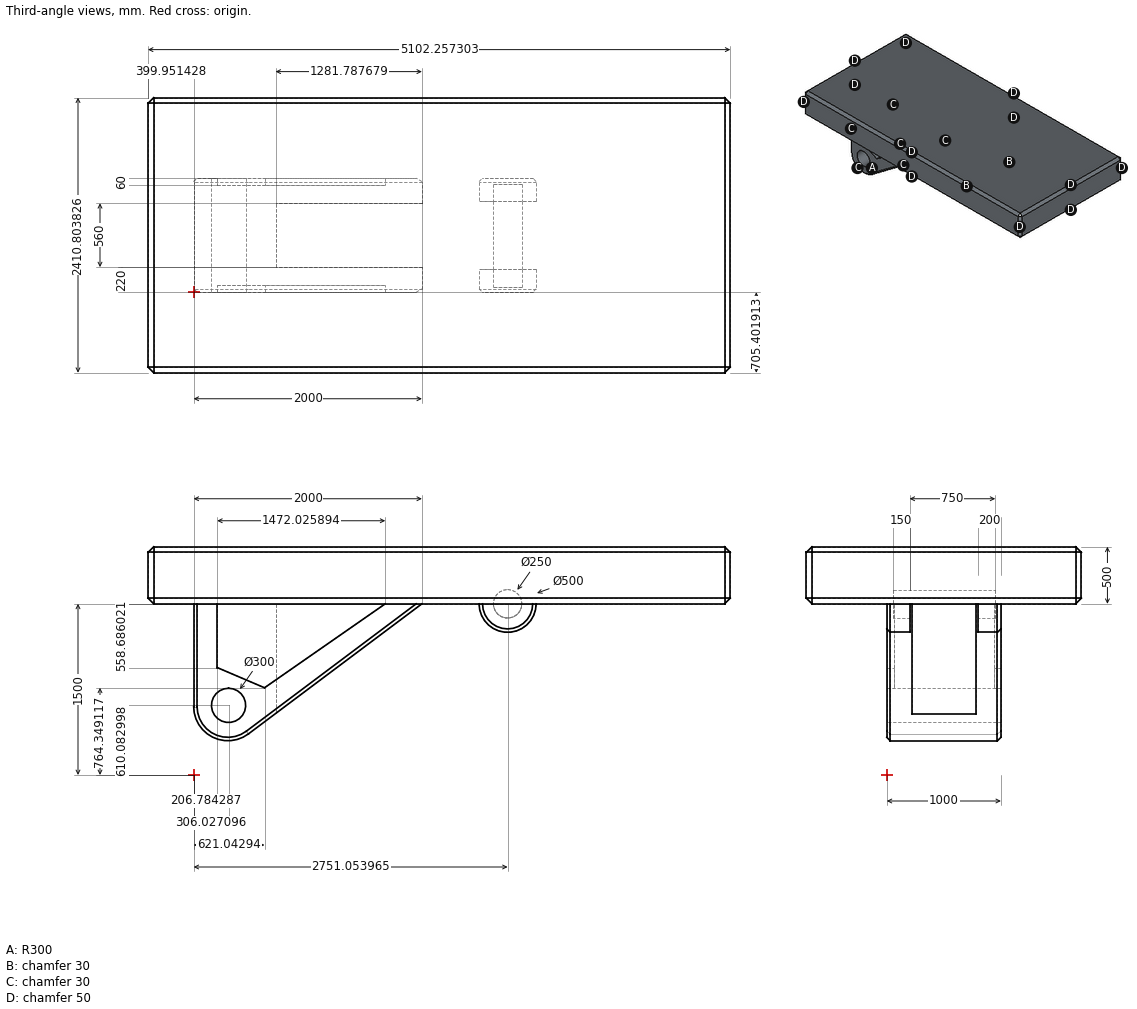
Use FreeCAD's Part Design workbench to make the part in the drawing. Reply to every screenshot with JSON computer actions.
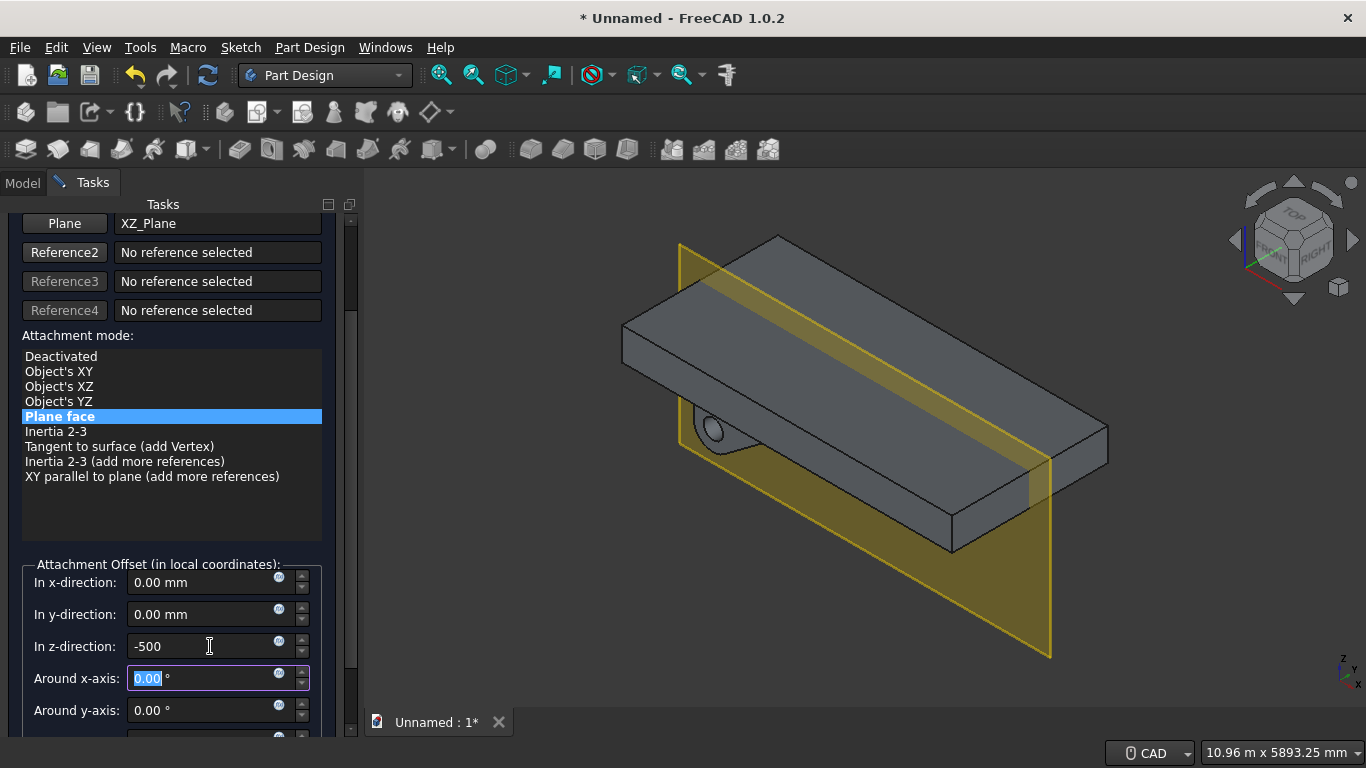
{"action": "scroll", "coordinate": [351, 475], "scroll_direction": "up", "scroll_amount": 3}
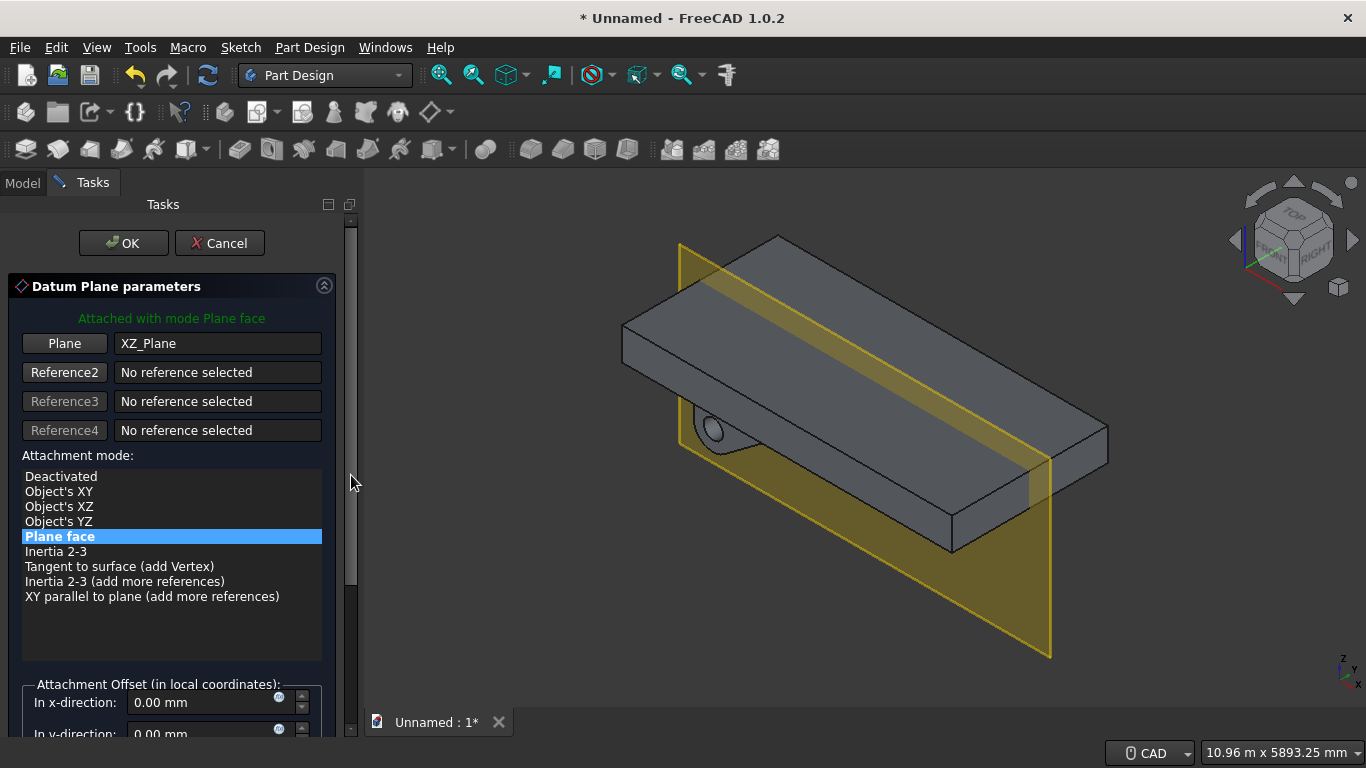
{"action": "left_click", "coordinate": [124, 243]}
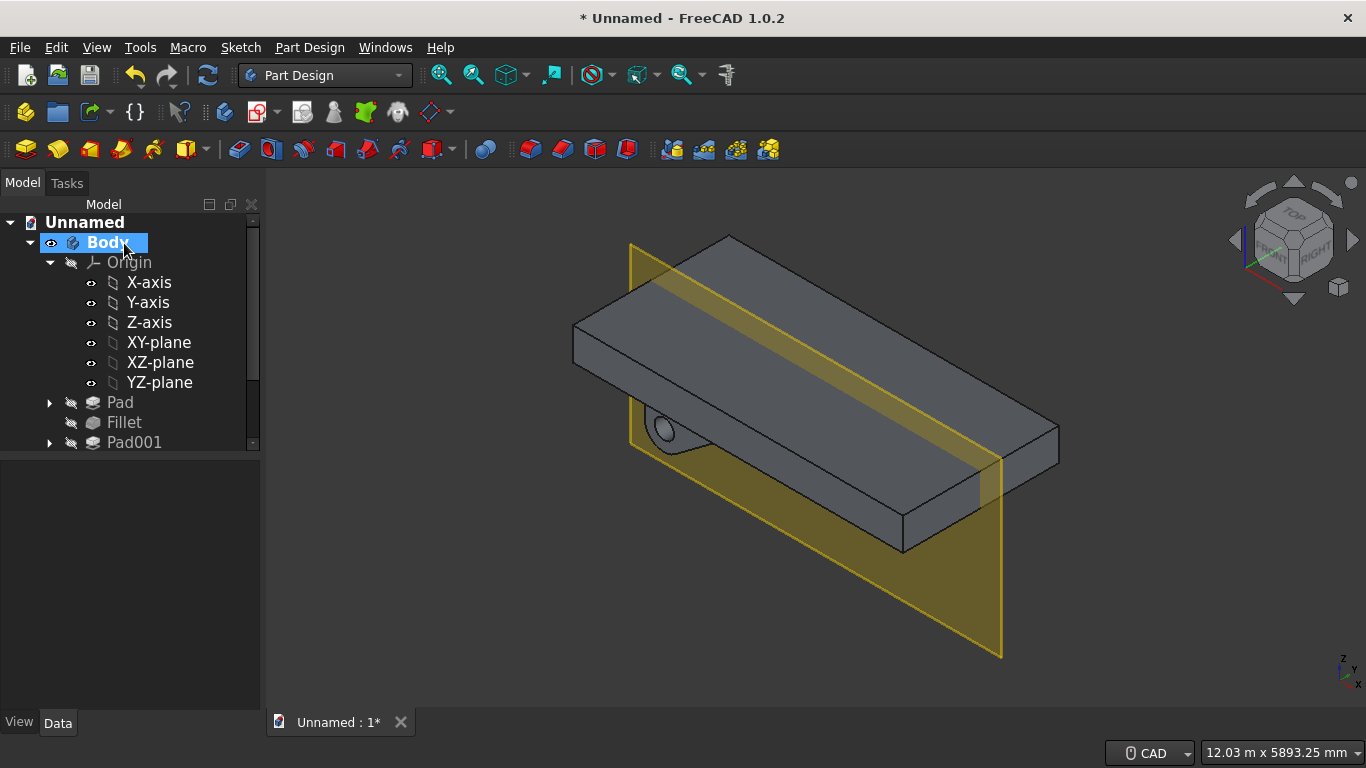
{"action": "scroll", "coordinate": [100, 338], "scroll_direction": "down", "scroll_amount": 3}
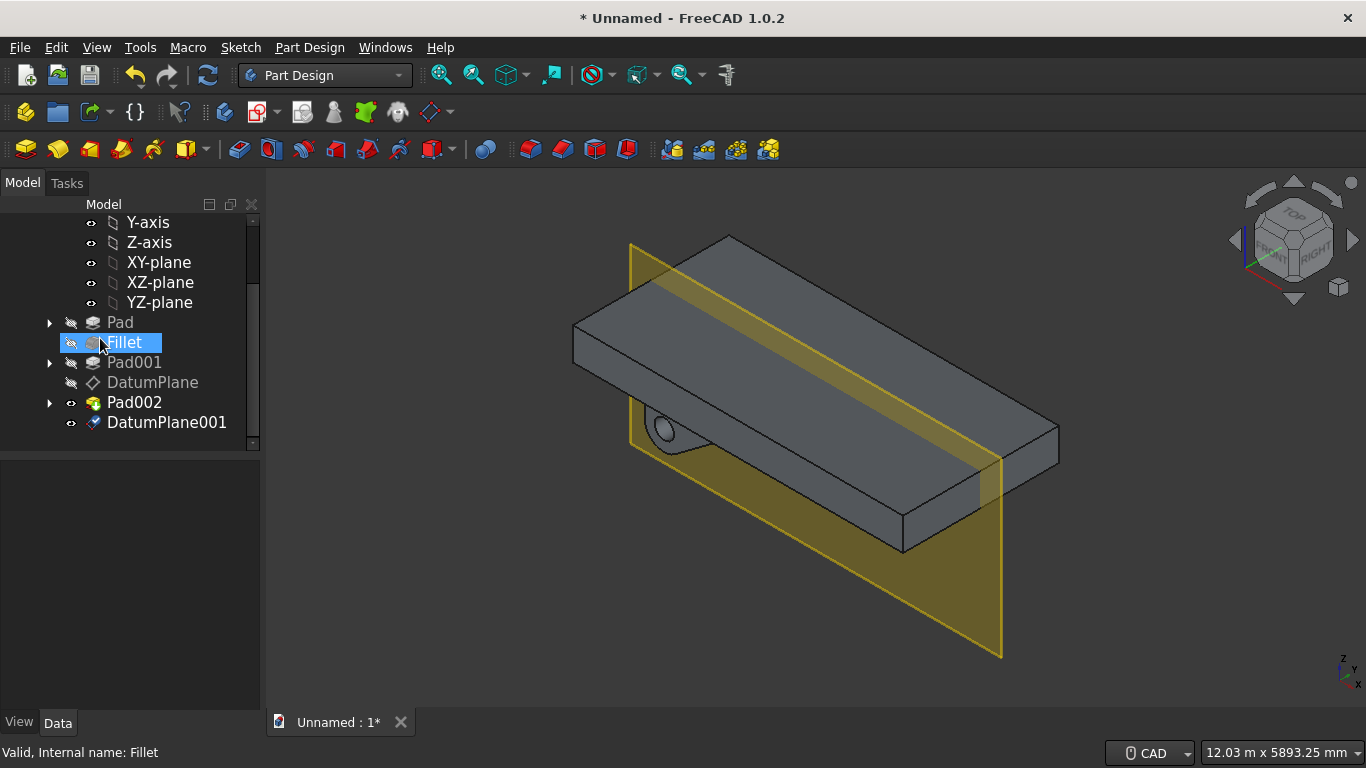
{"action": "left_click", "coordinate": [116, 403]}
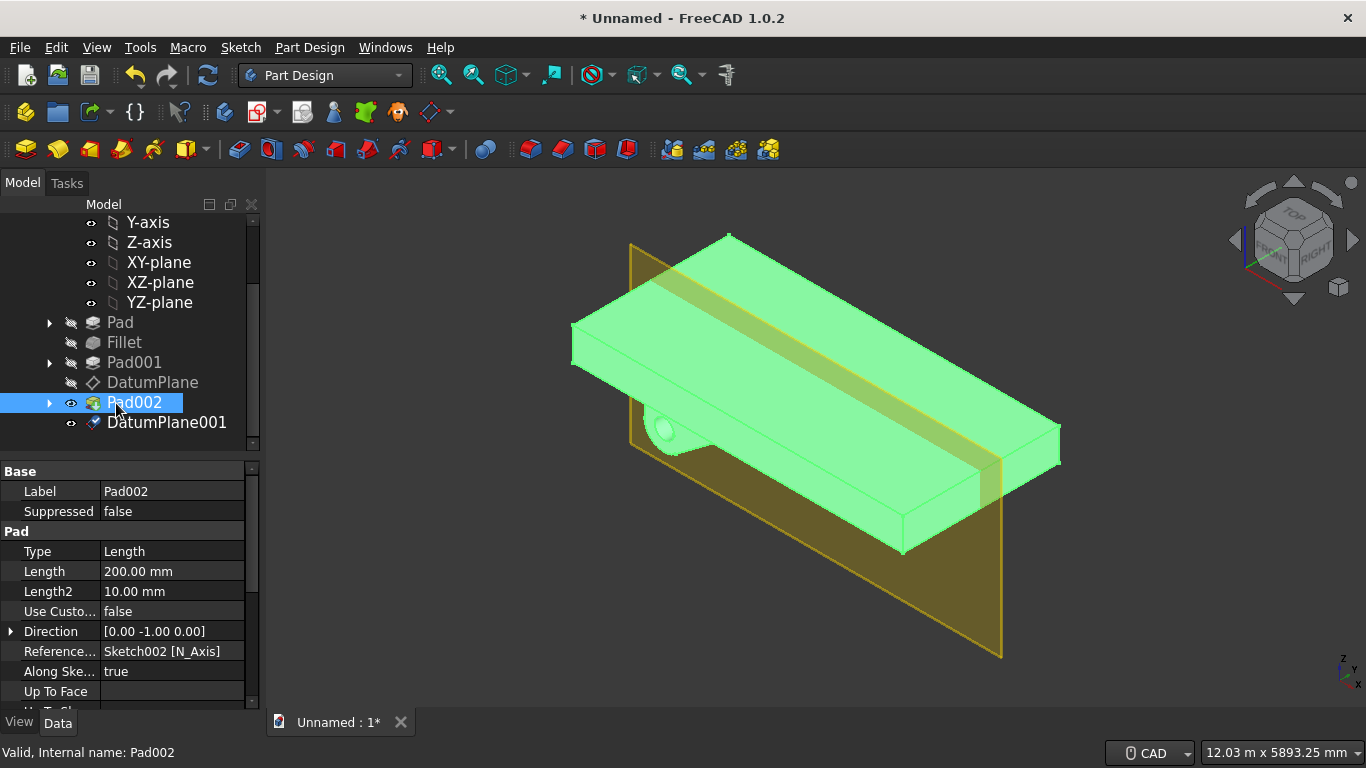
{"action": "left_click", "coordinate": [672, 150]}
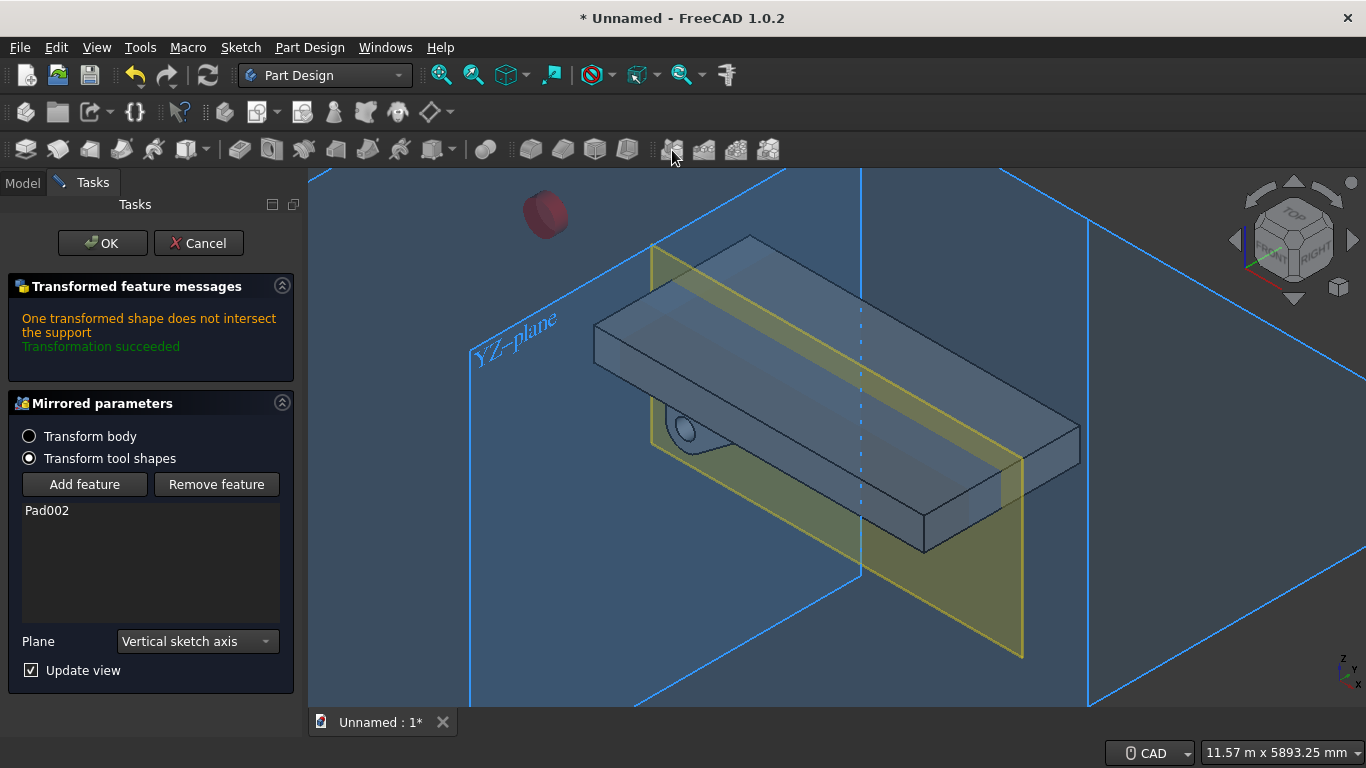
{"action": "left_click", "coordinate": [198, 642]}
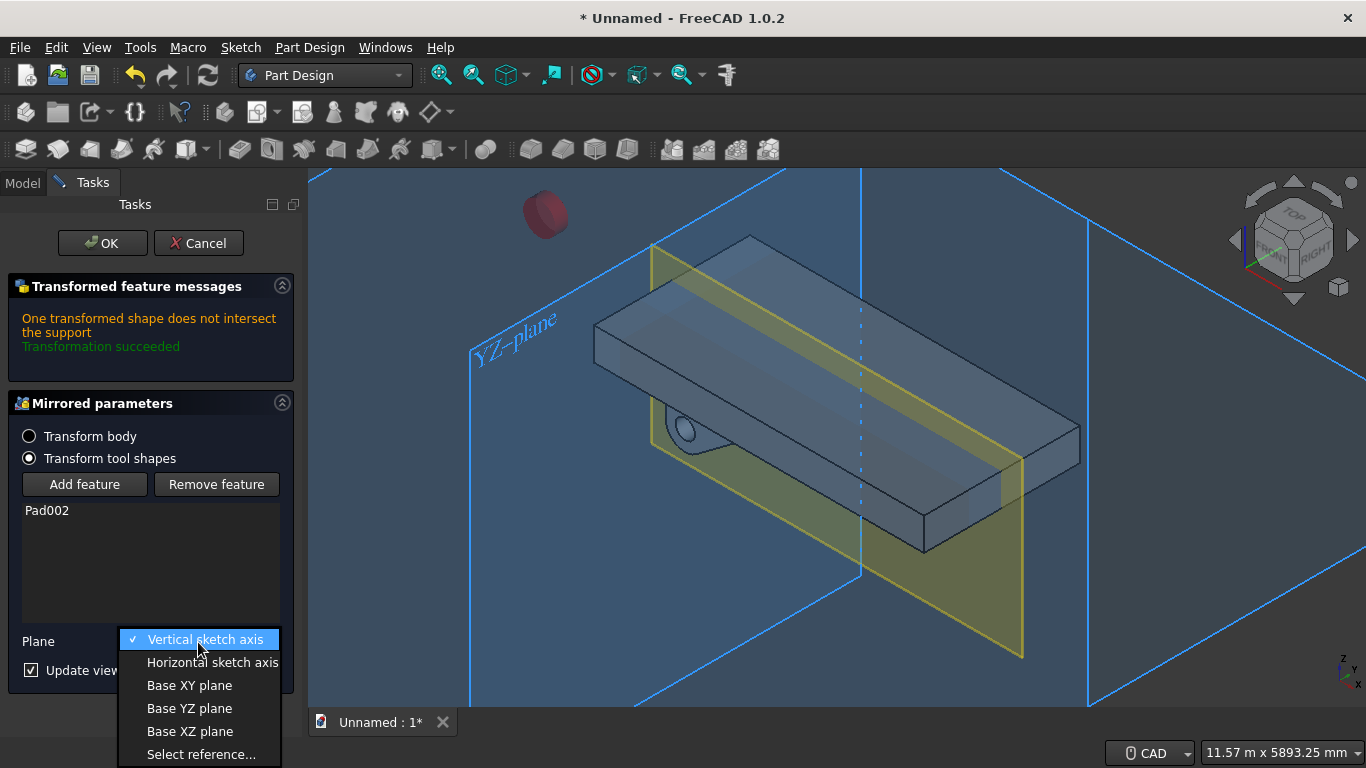
{"action": "left_click", "coordinate": [198, 754]}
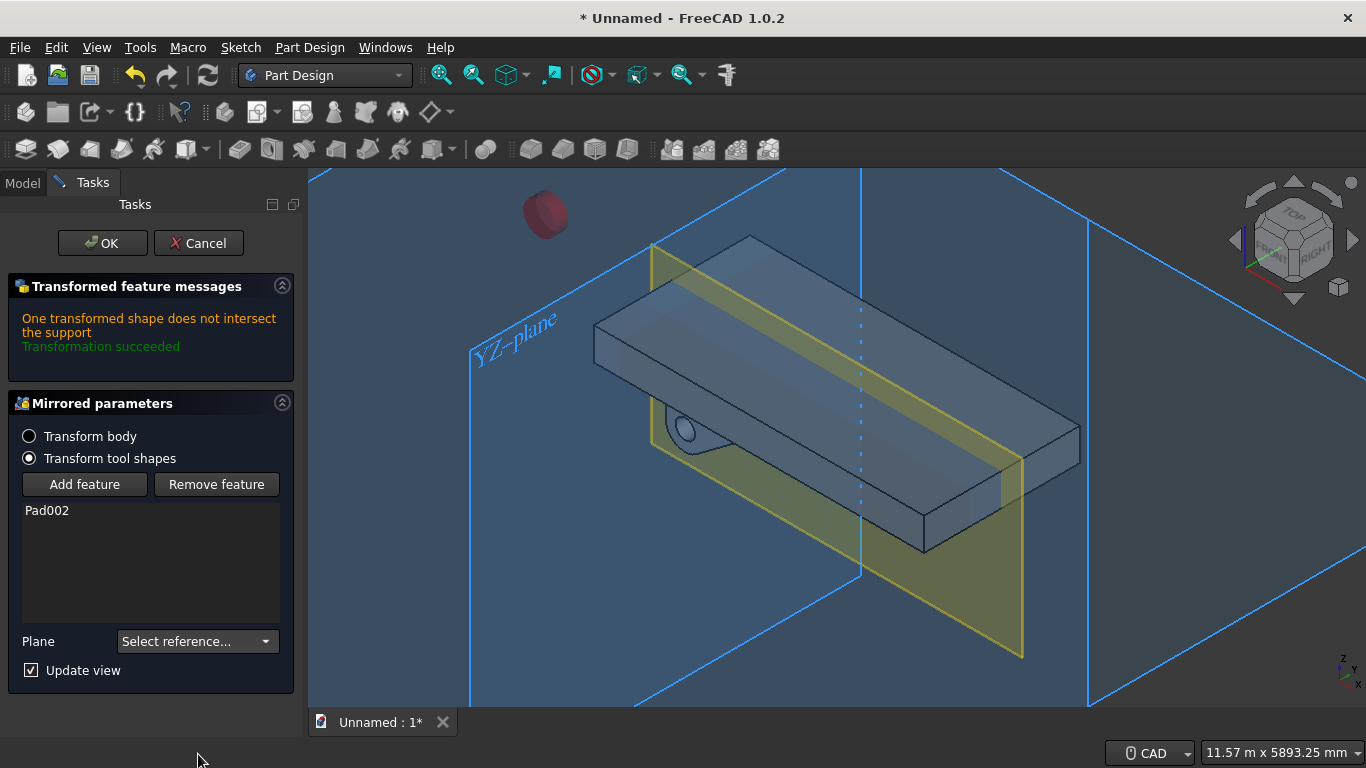
{"action": "left_click", "coordinate": [23, 182]}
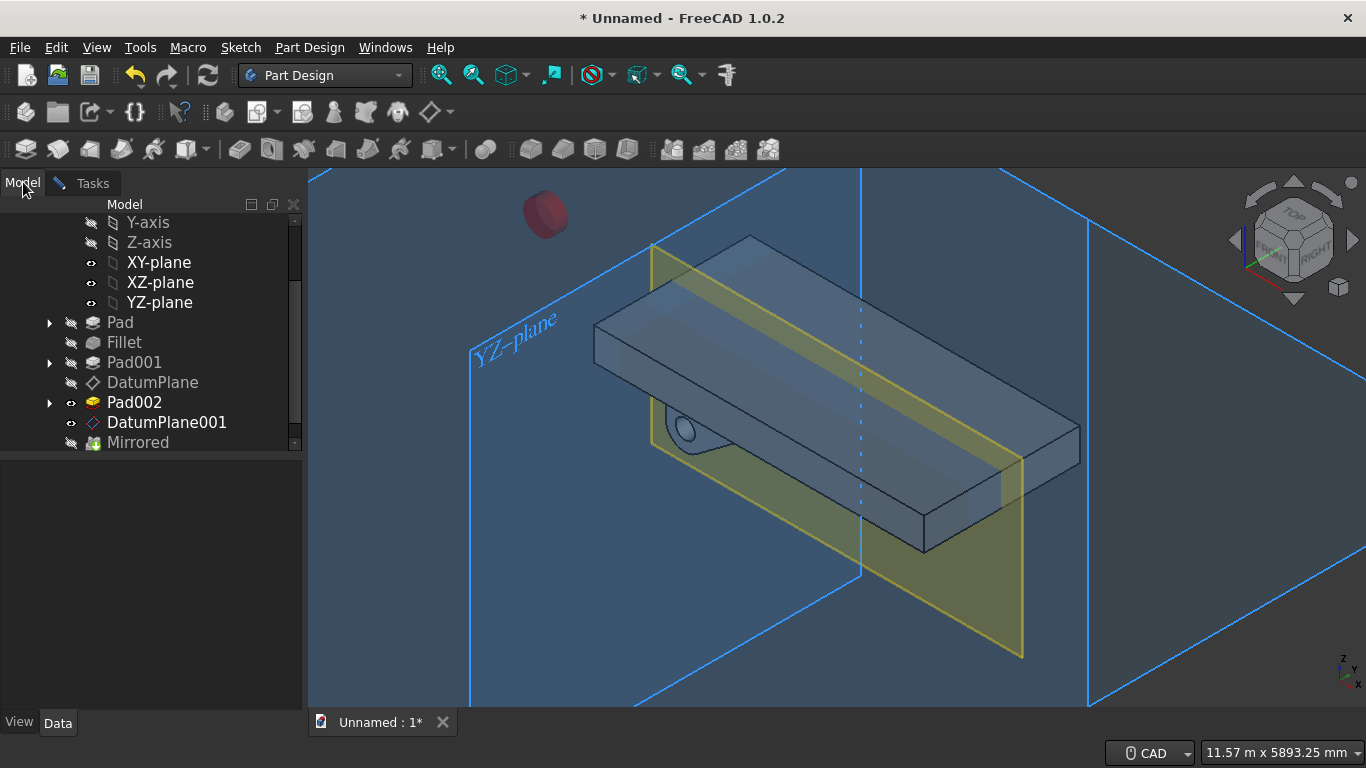
{"action": "left_click", "coordinate": [116, 423]}